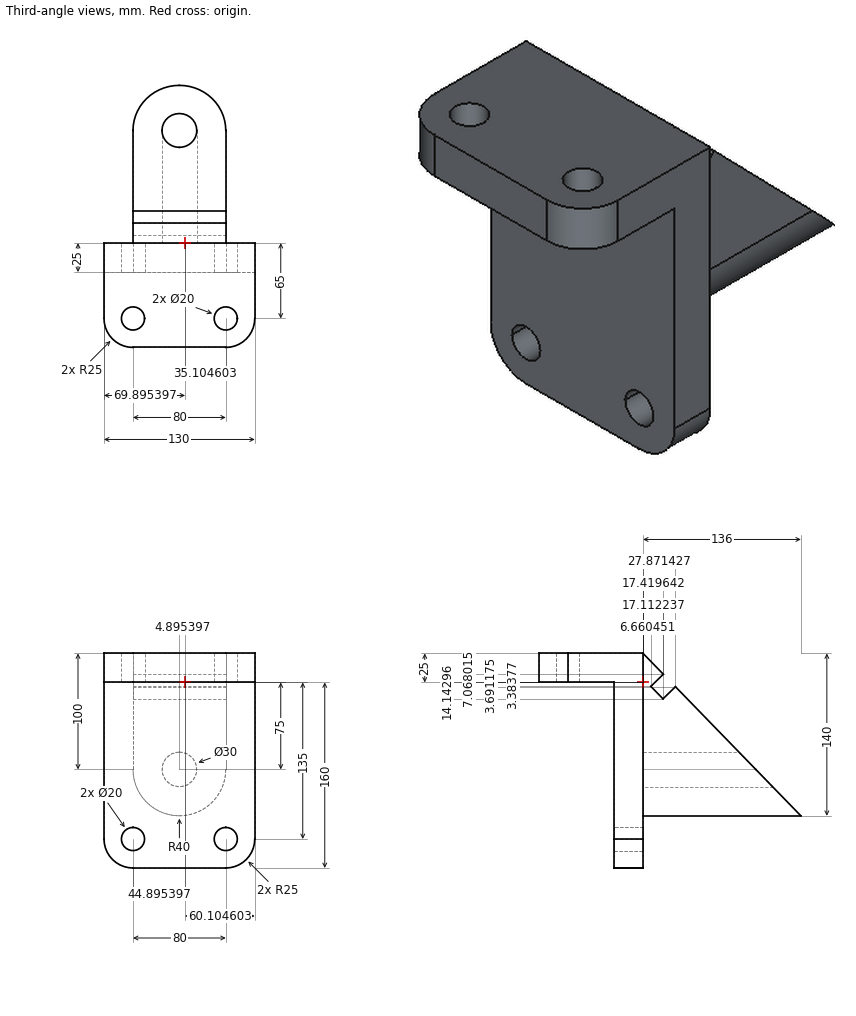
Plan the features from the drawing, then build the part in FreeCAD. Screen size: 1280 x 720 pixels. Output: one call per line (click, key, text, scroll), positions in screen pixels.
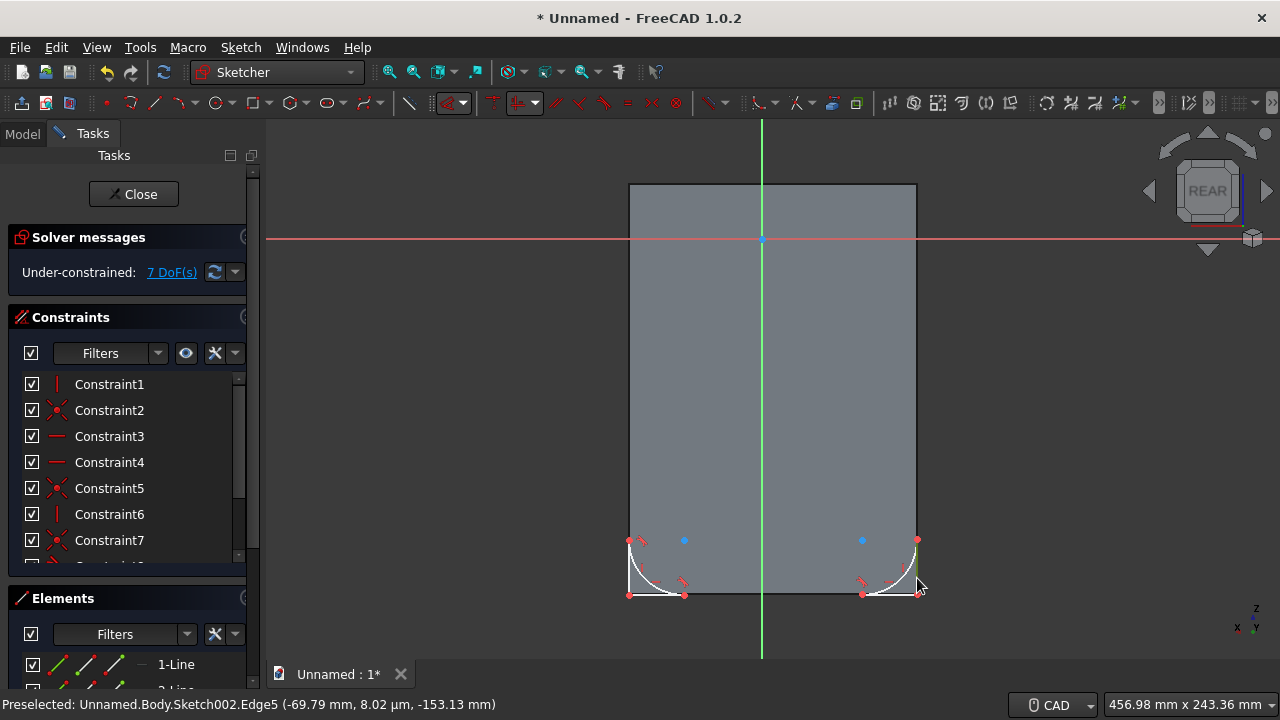
click(901, 579)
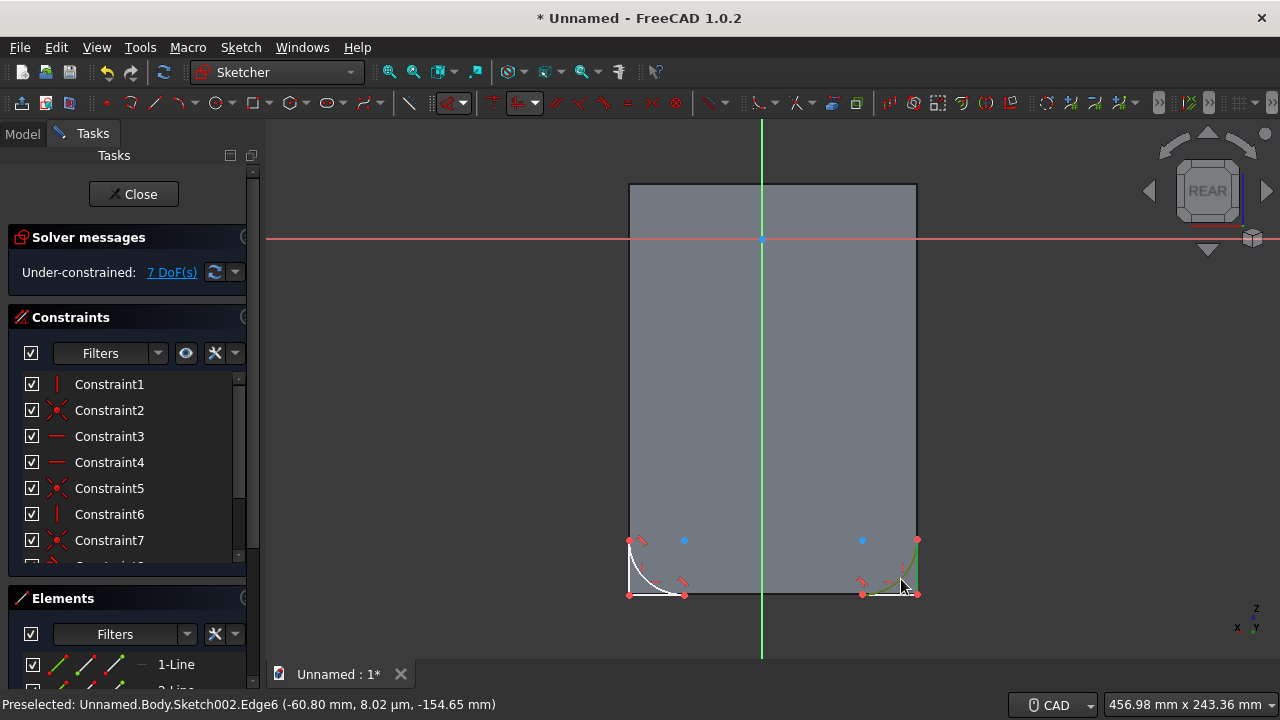
key(t)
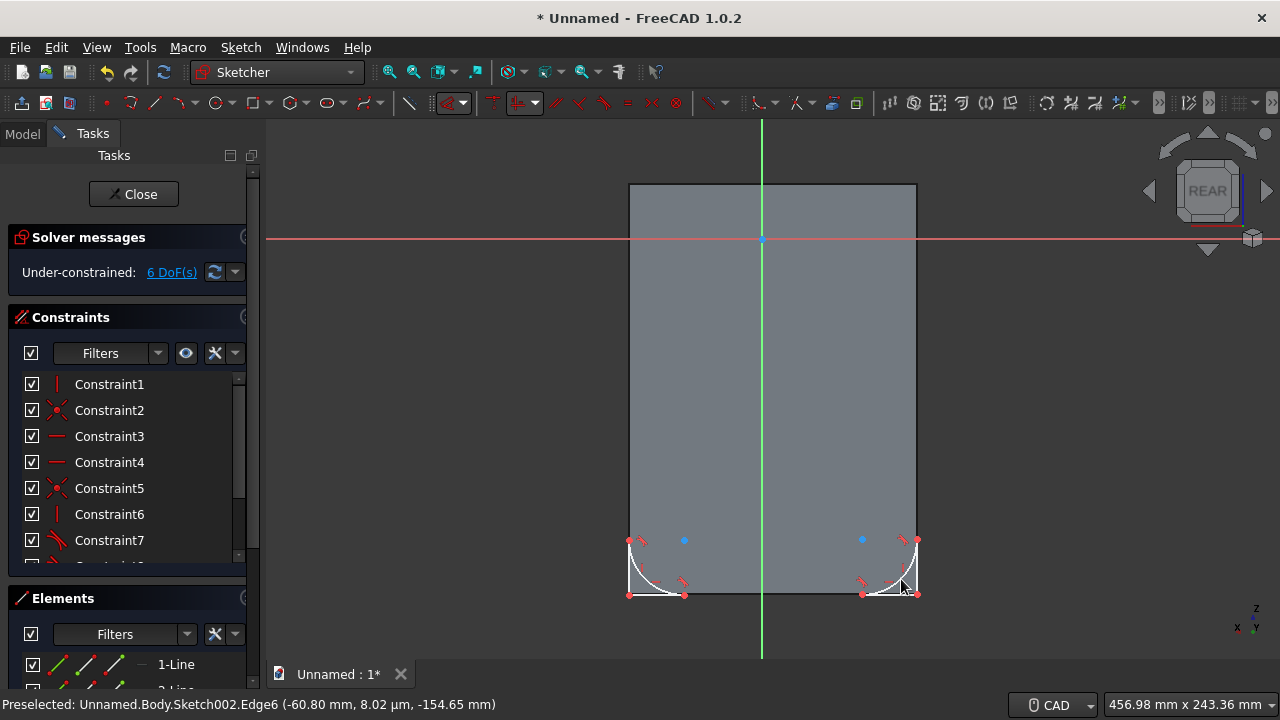
click(645, 579)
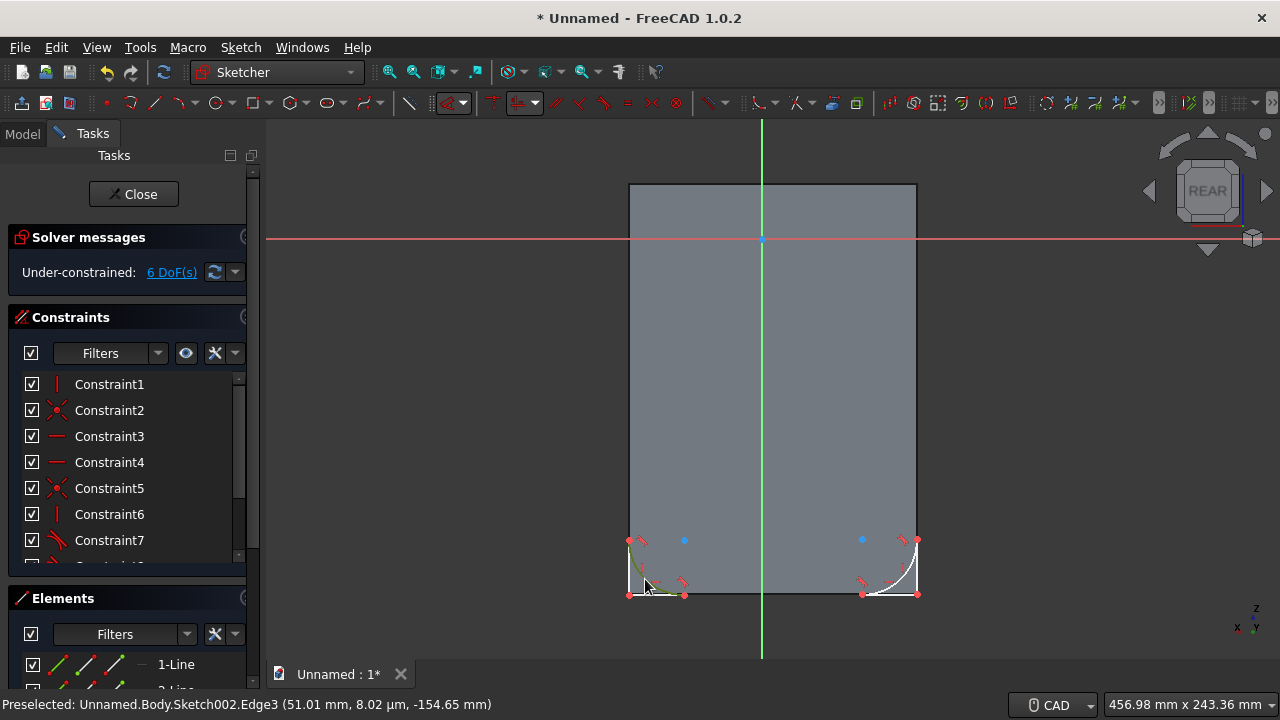
click(901, 579)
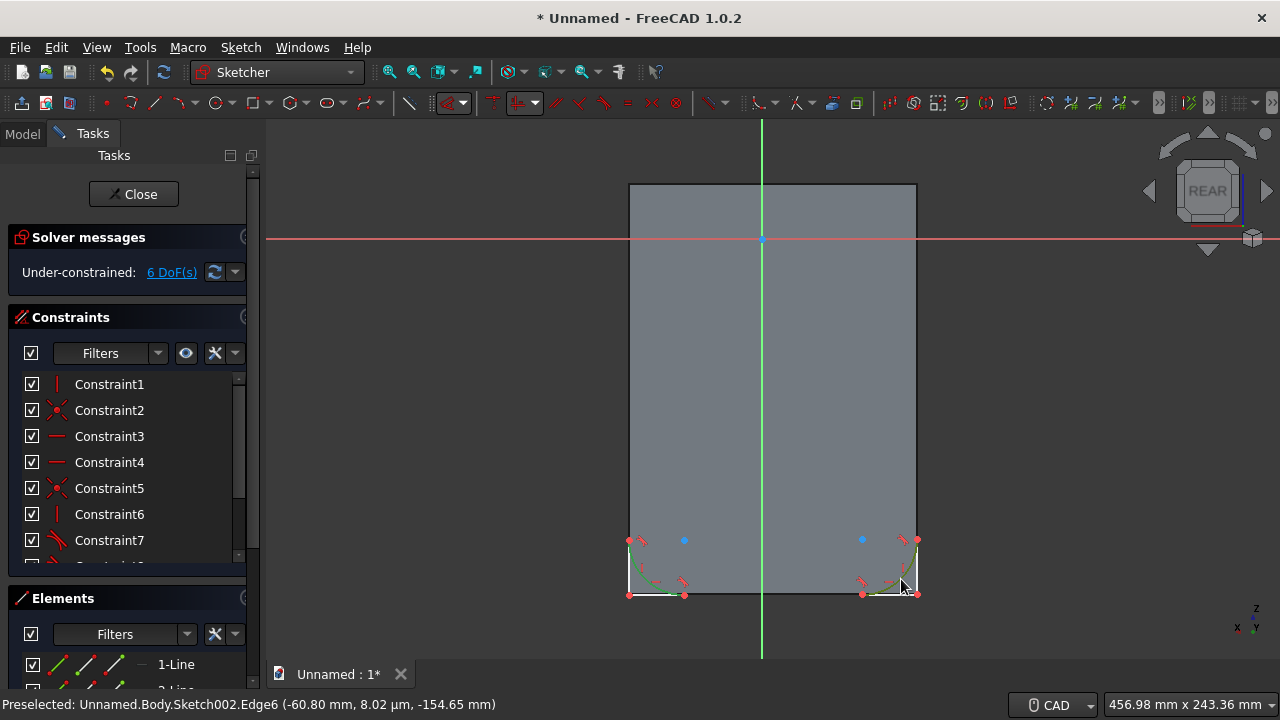
click(628, 104)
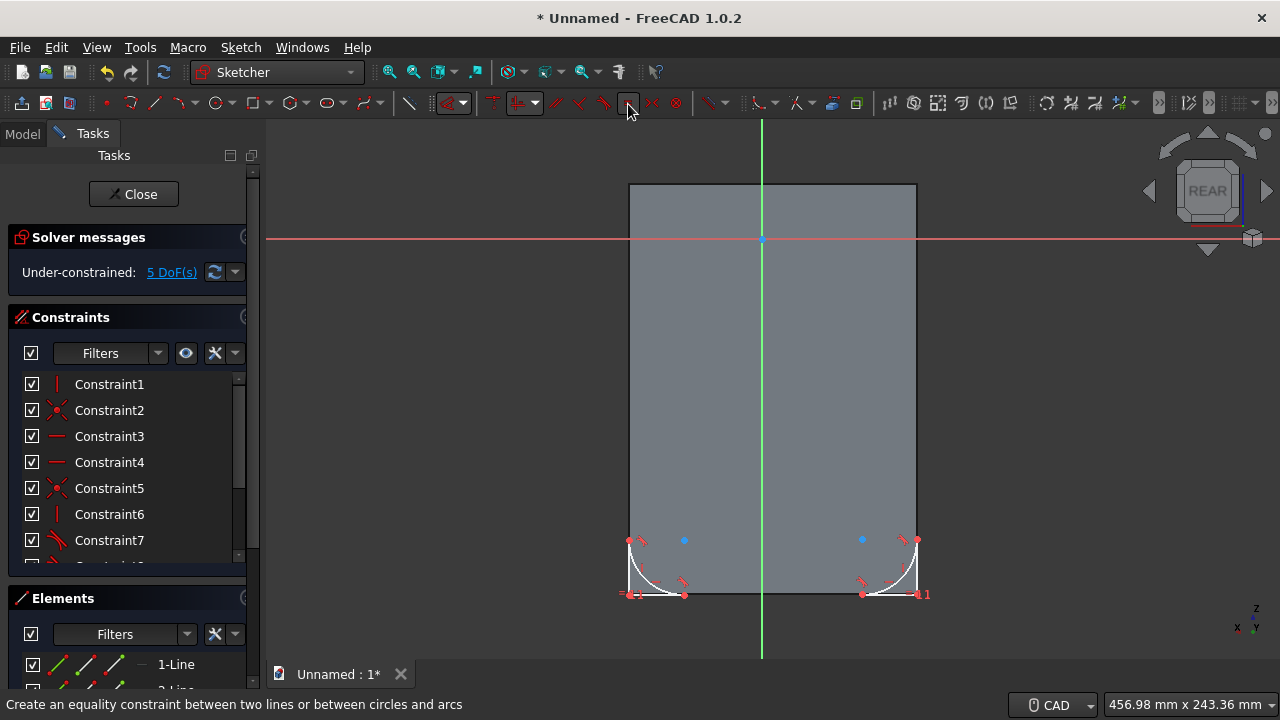
click(645, 579)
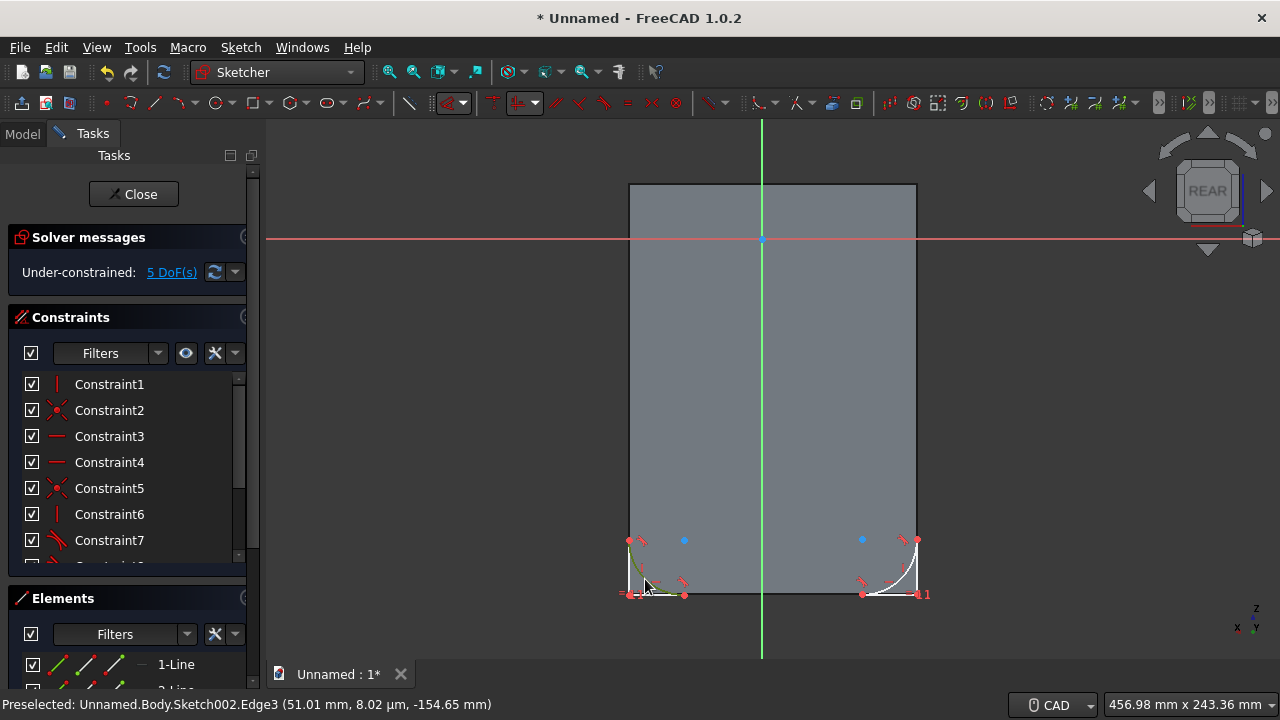
key(k)
key(r)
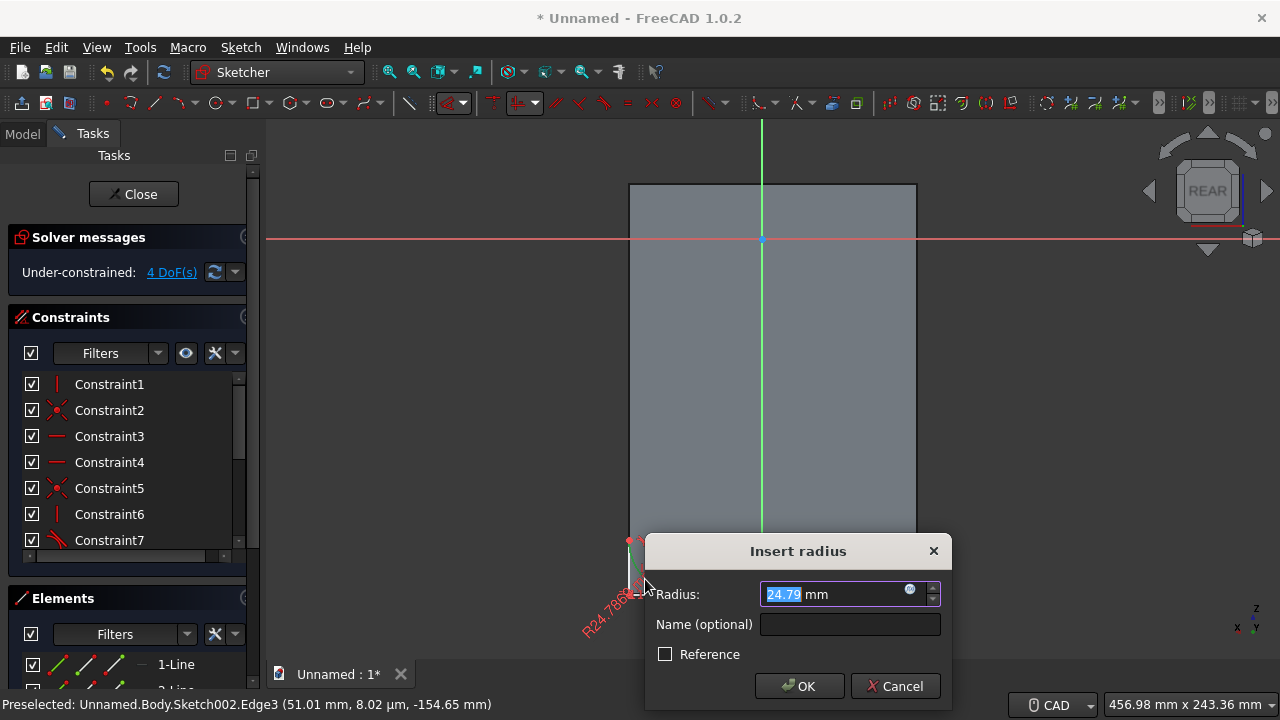
text(25)
key(Return)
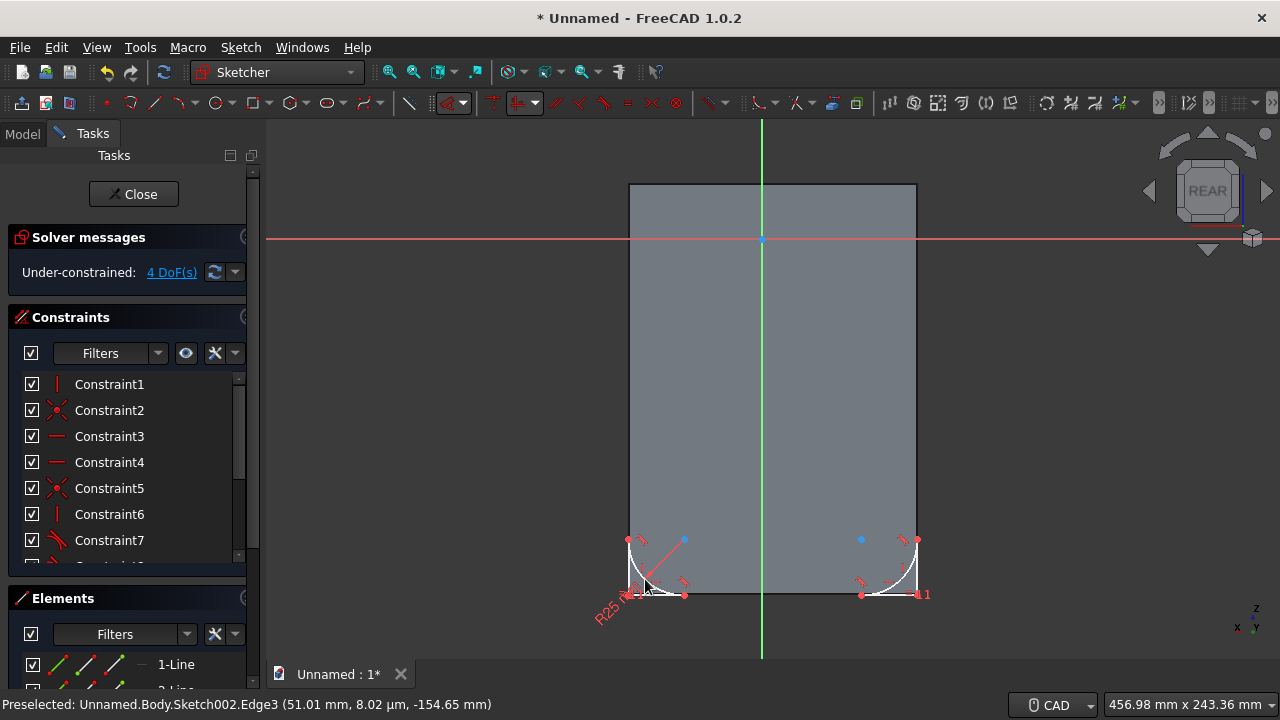
click(629, 540)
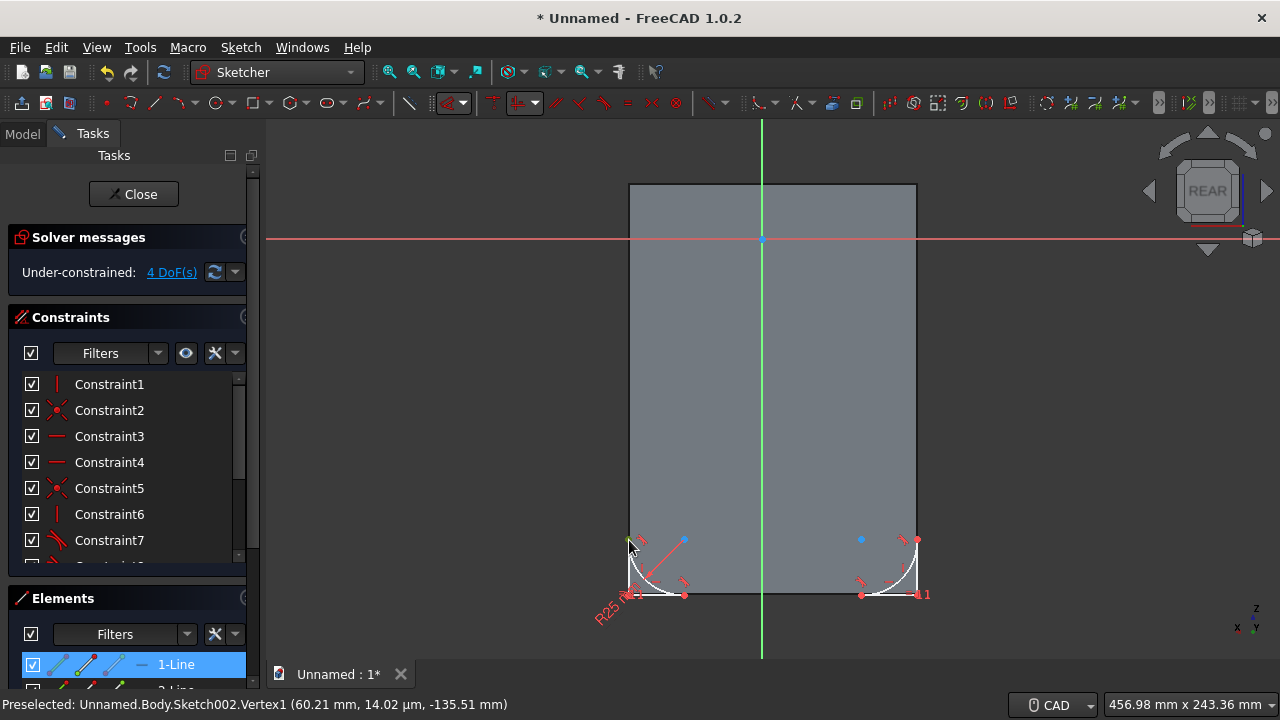
key(i)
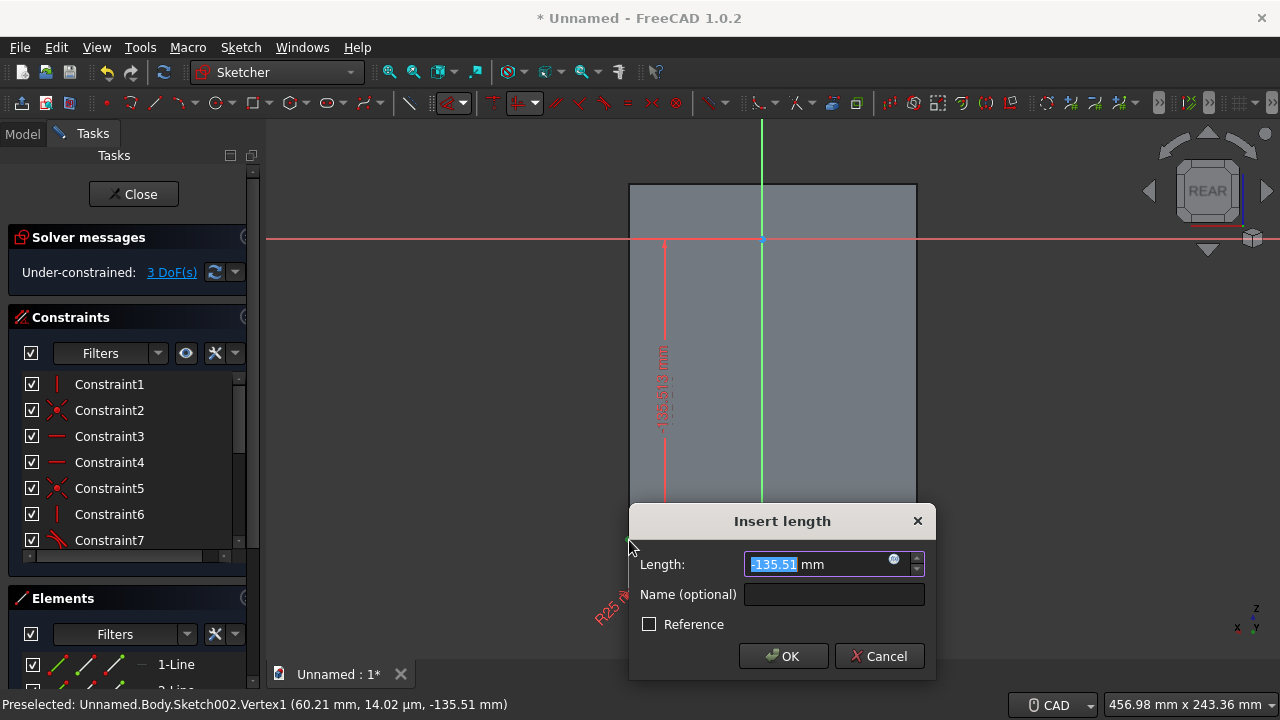
text(-135)
key(Return)